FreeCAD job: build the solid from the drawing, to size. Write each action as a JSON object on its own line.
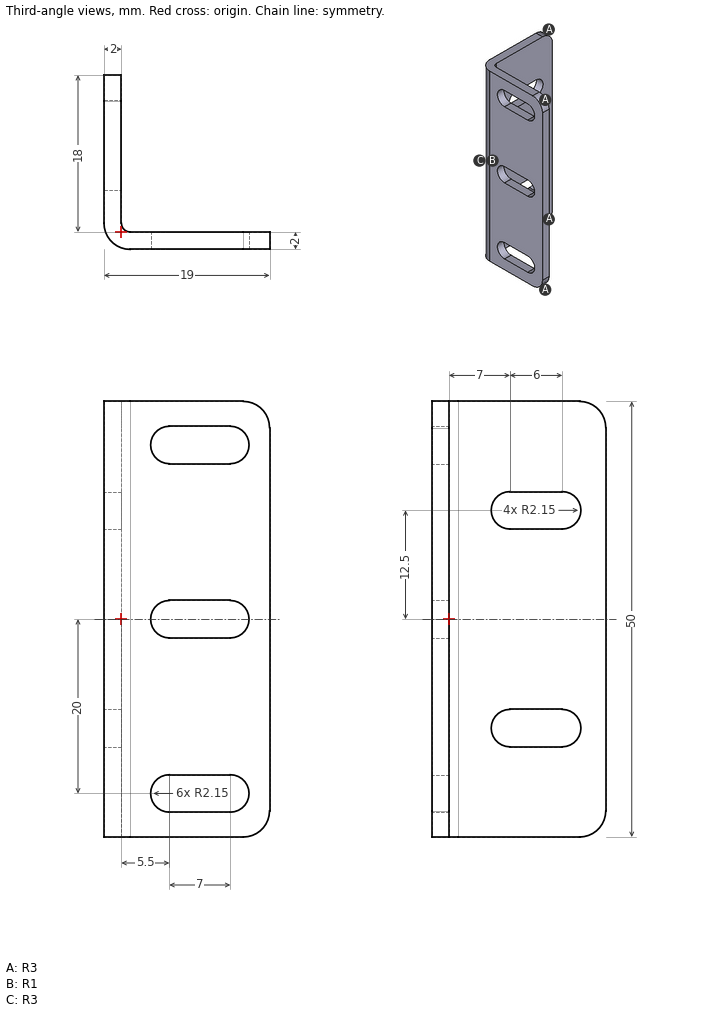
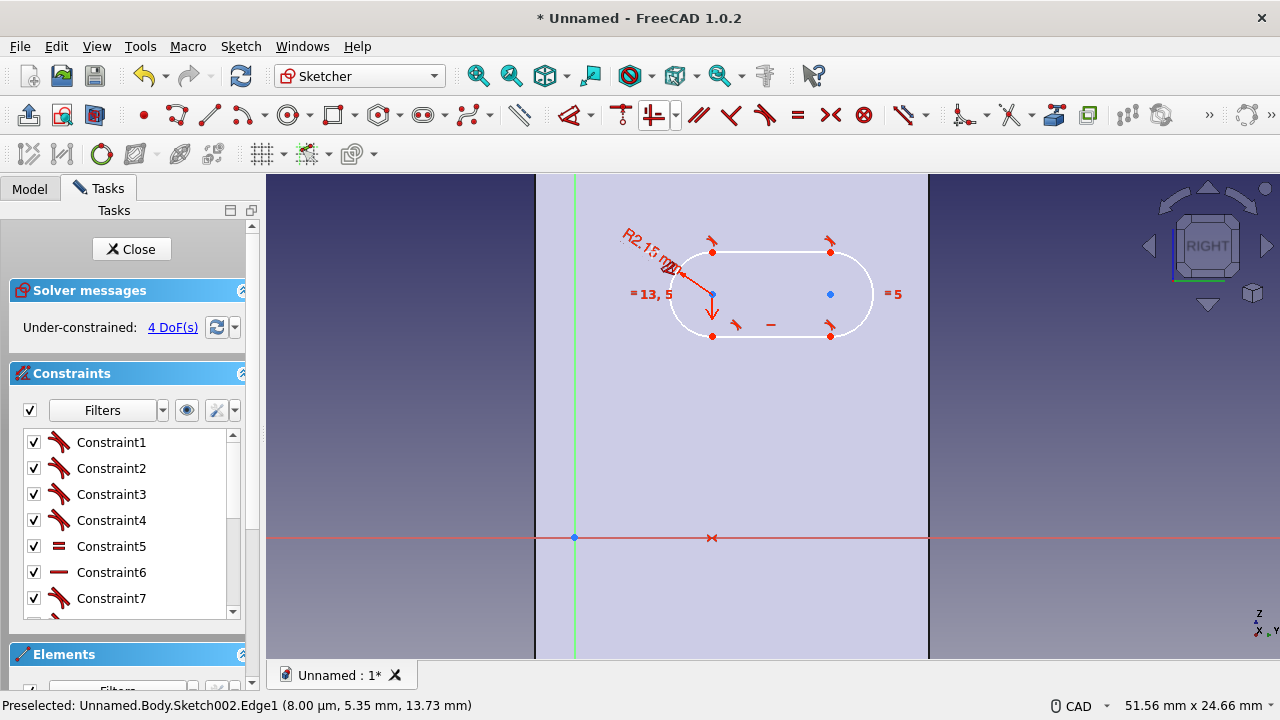
{"action": "left_click", "coordinate": [748, 252]}
{"action": "left_click", "coordinate": [772, 218]}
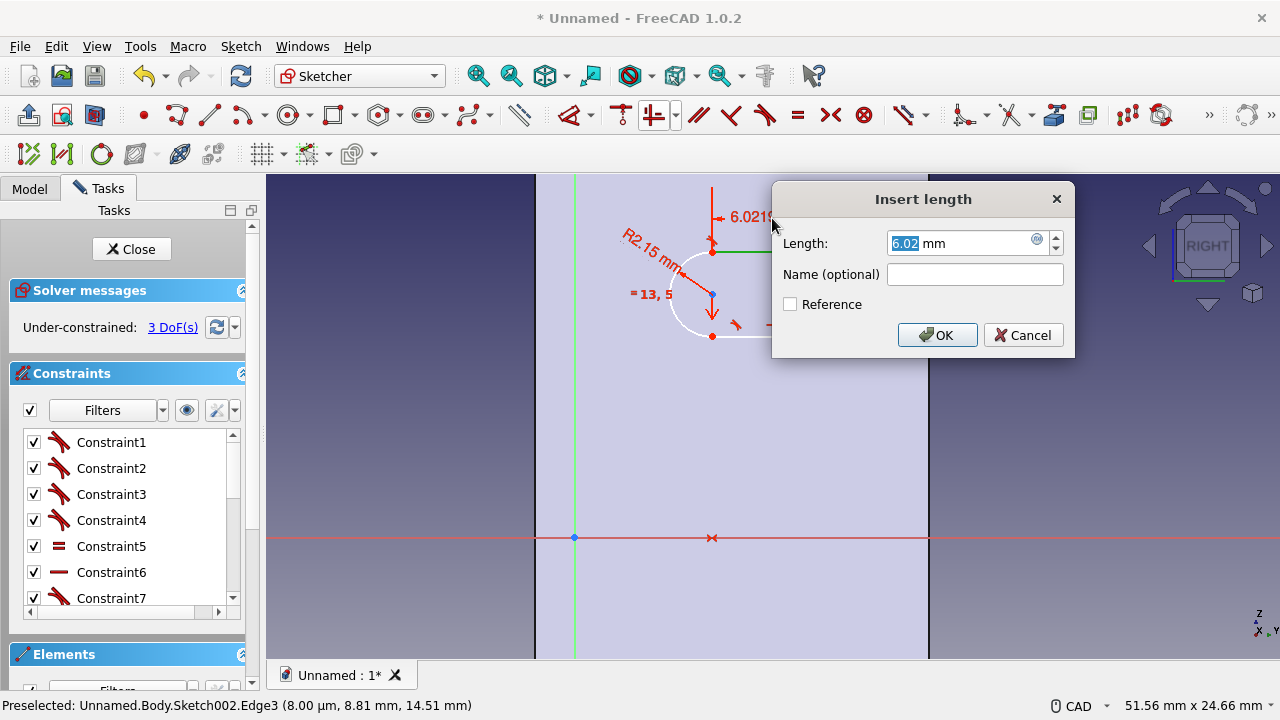
{"action": "type", "text": "6"}
{"action": "key", "text": "Return"}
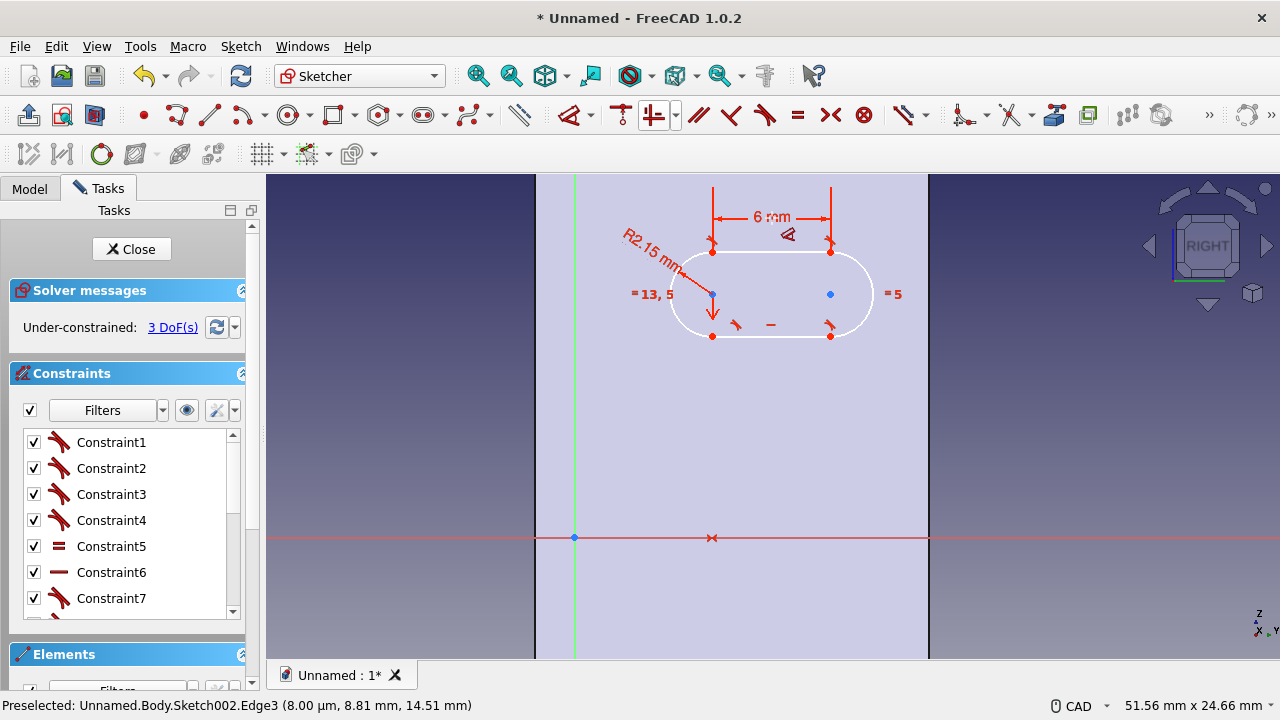
{"action": "scroll", "coordinate": [681, 269], "scroll_direction": "down", "scroll_amount": 3}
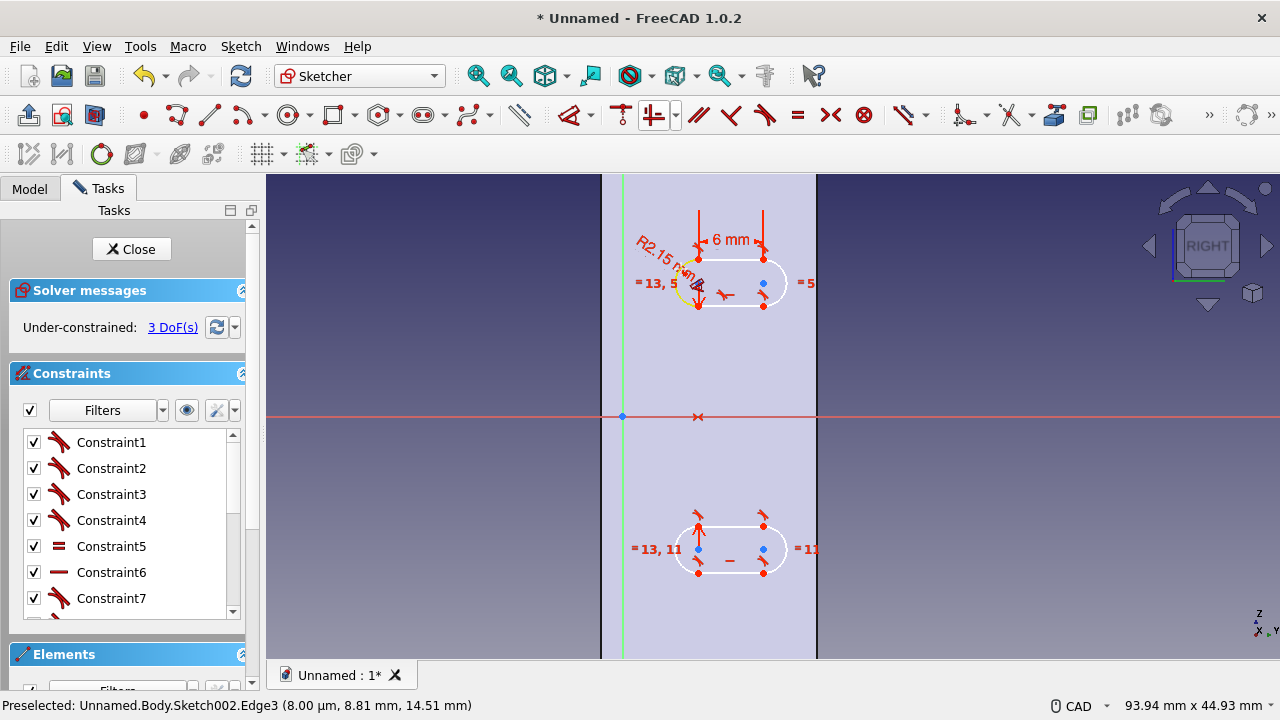
{"action": "left_click", "coordinate": [718, 527]}
{"action": "left_click", "coordinate": [731, 493]}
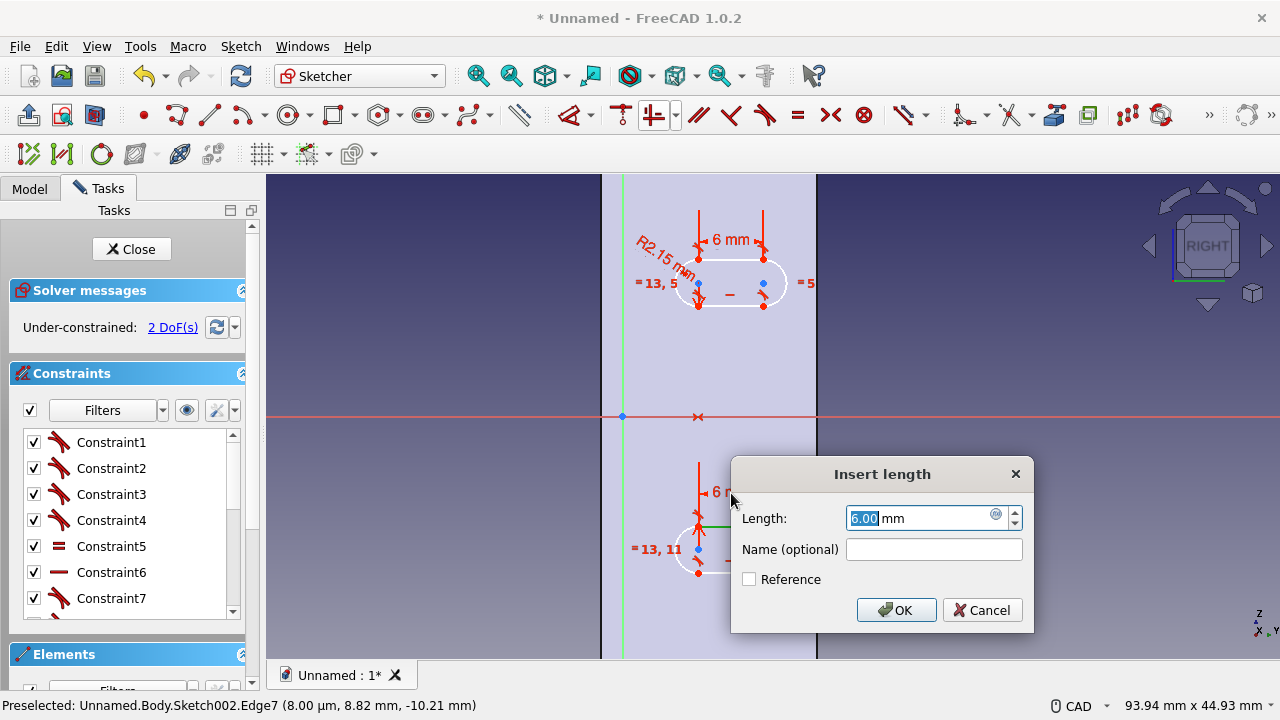
{"action": "type", "text": "6"}
{"action": "key", "text": "Return"}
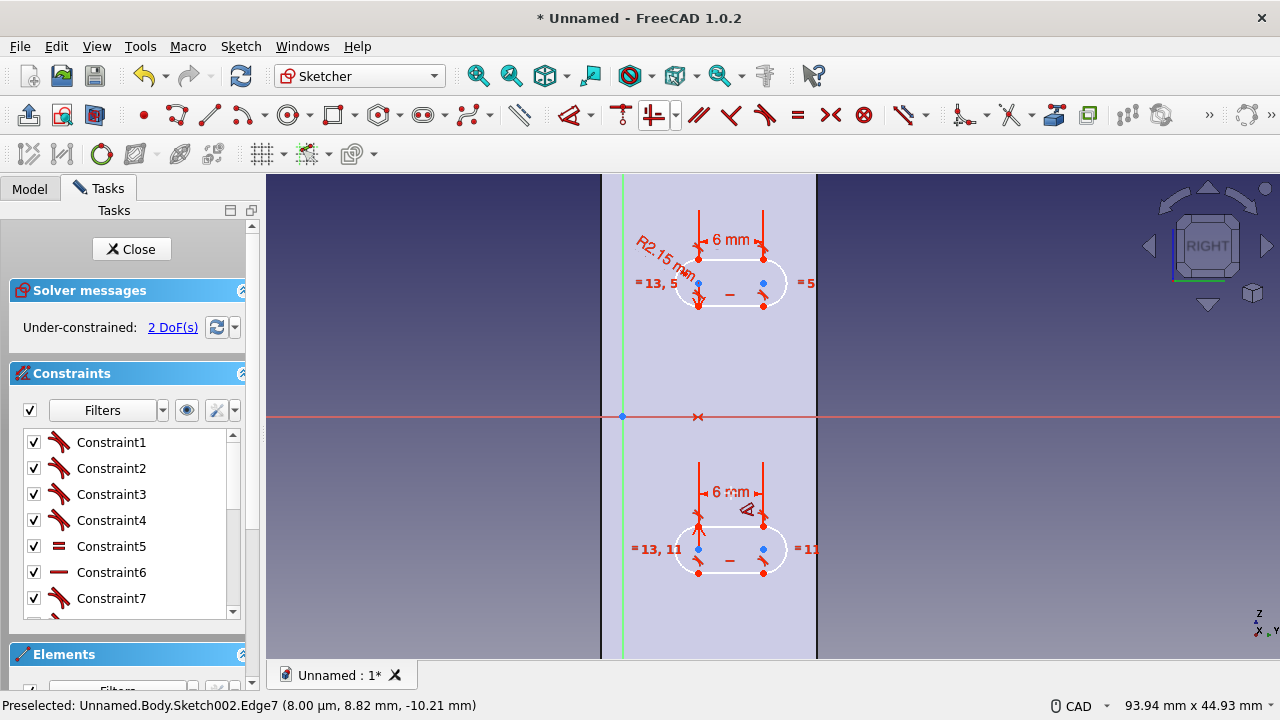
{"action": "left_click", "coordinate": [699, 260]}
{"action": "left_click", "coordinate": [661, 226]}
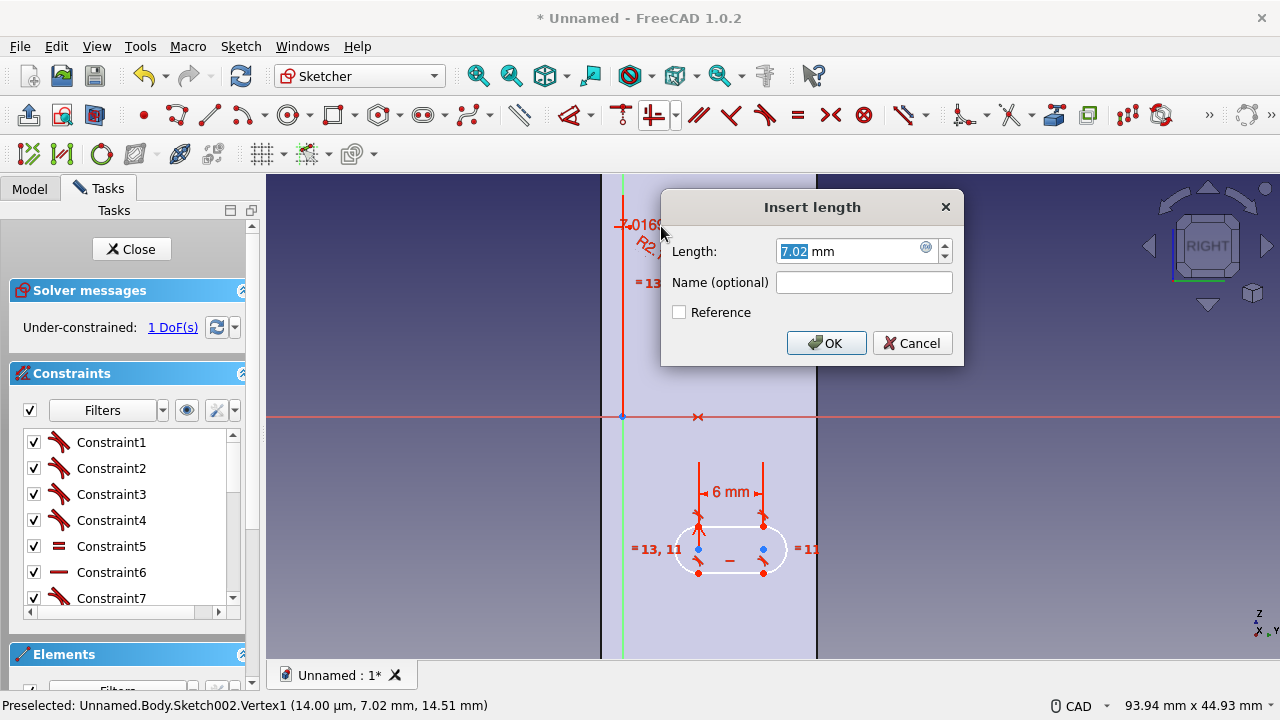
{"action": "type", "text": "7"}
{"action": "key", "text": "Return"}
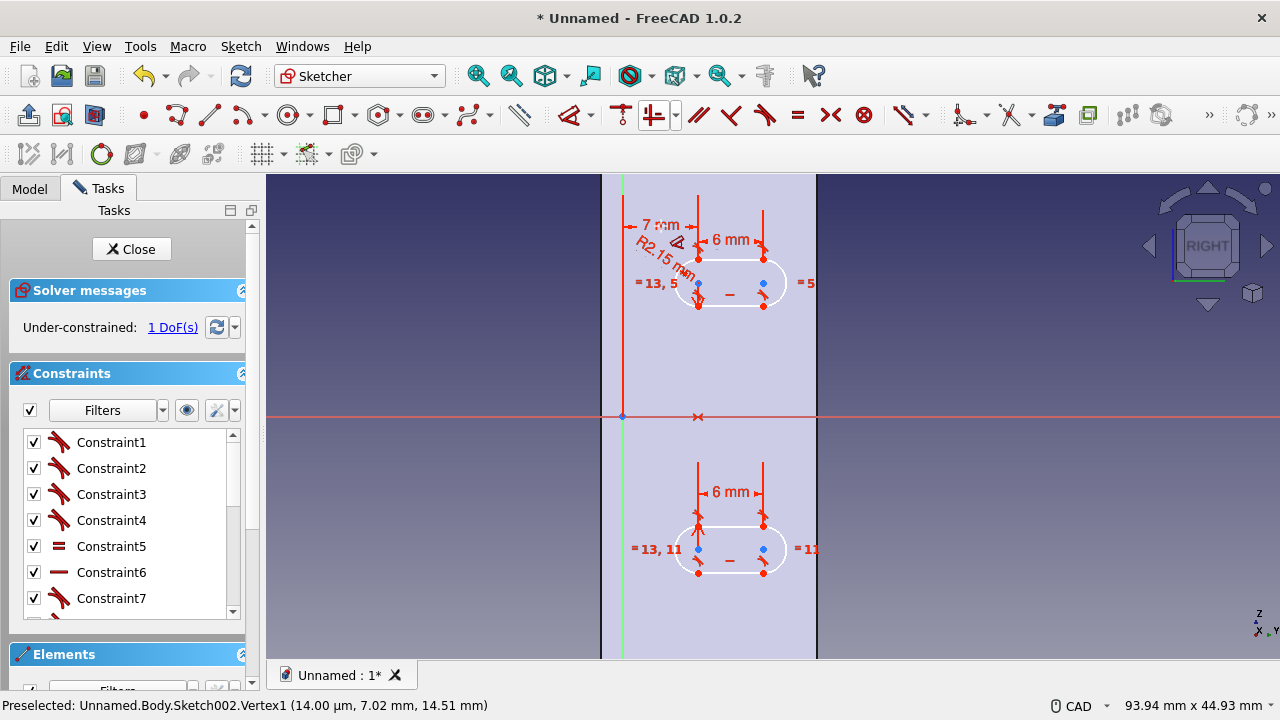
{"action": "left_click", "coordinate": [698, 283]}
{"action": "left_click", "coordinate": [589, 350]}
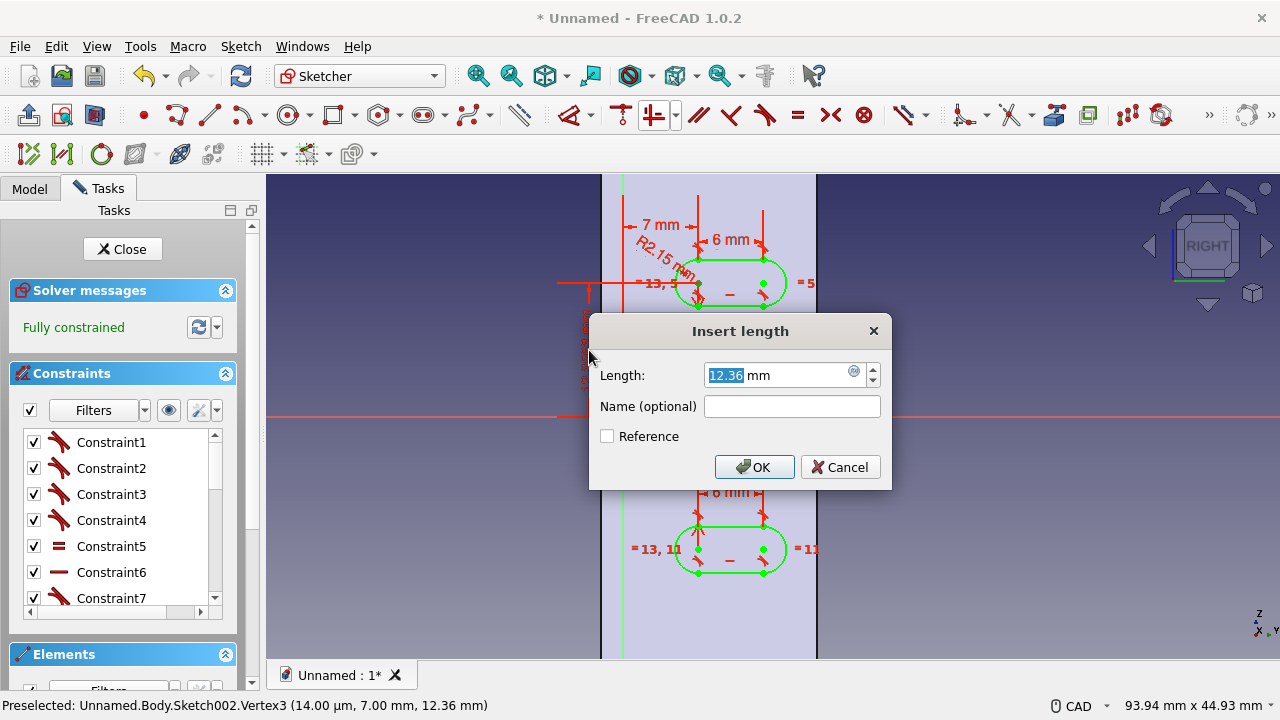
{"action": "type", "text": "12.5"}
{"action": "key", "text": "Return"}
{"action": "key", "text": "Escape"}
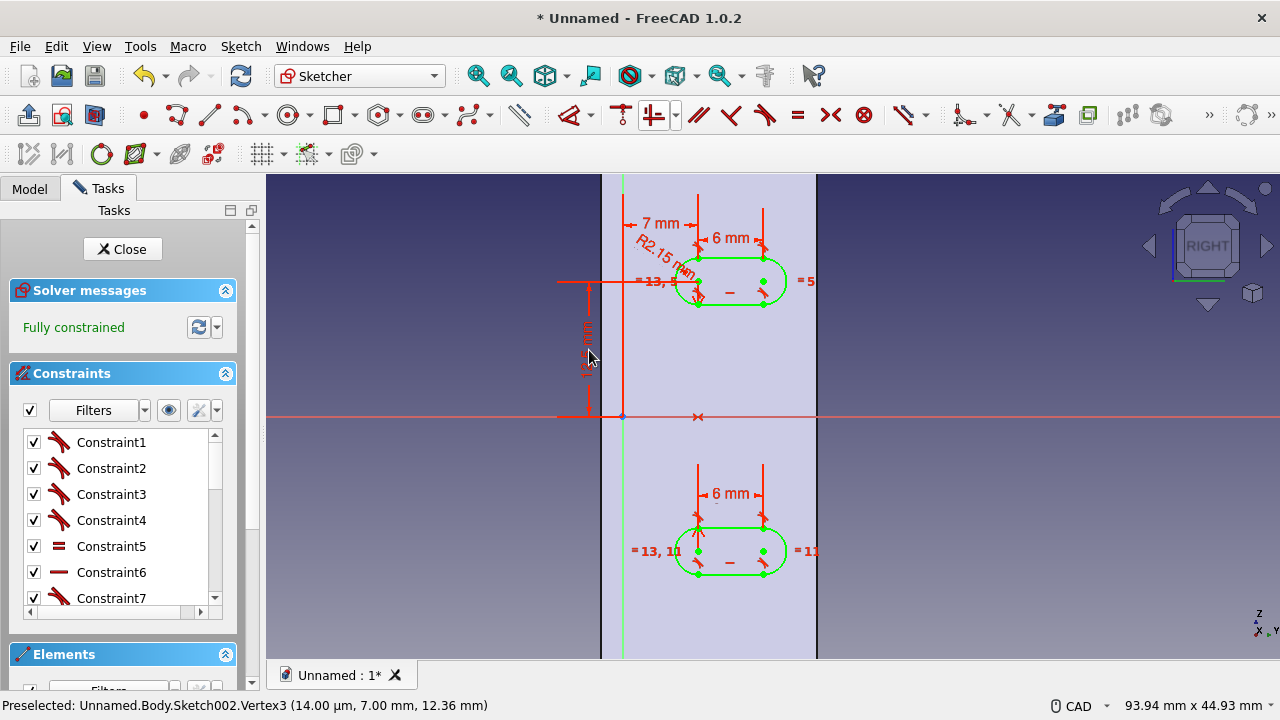
{"action": "left_click", "coordinate": [123, 249]}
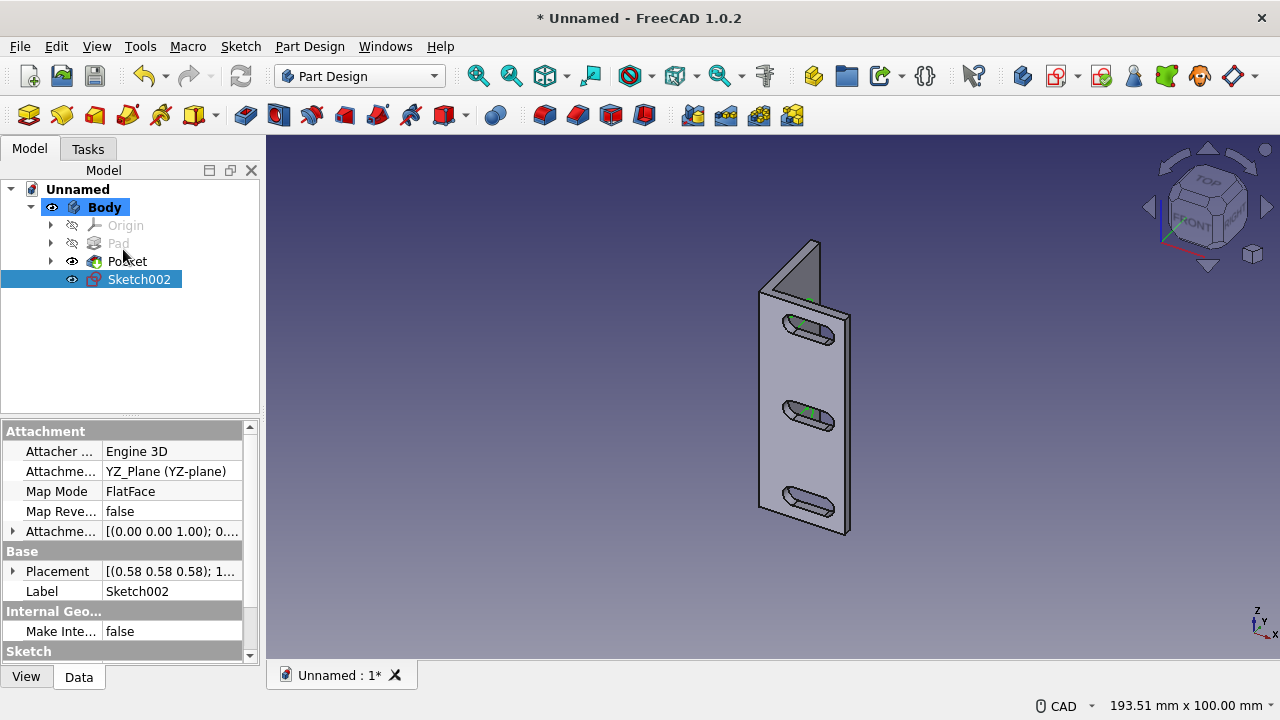
{"action": "left_click", "coordinate": [246, 116]}